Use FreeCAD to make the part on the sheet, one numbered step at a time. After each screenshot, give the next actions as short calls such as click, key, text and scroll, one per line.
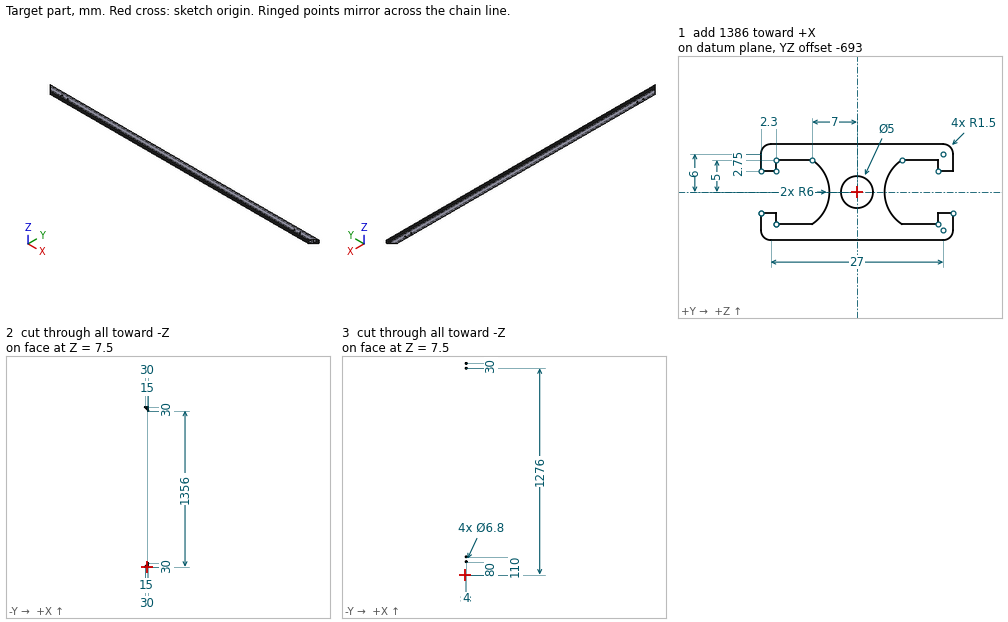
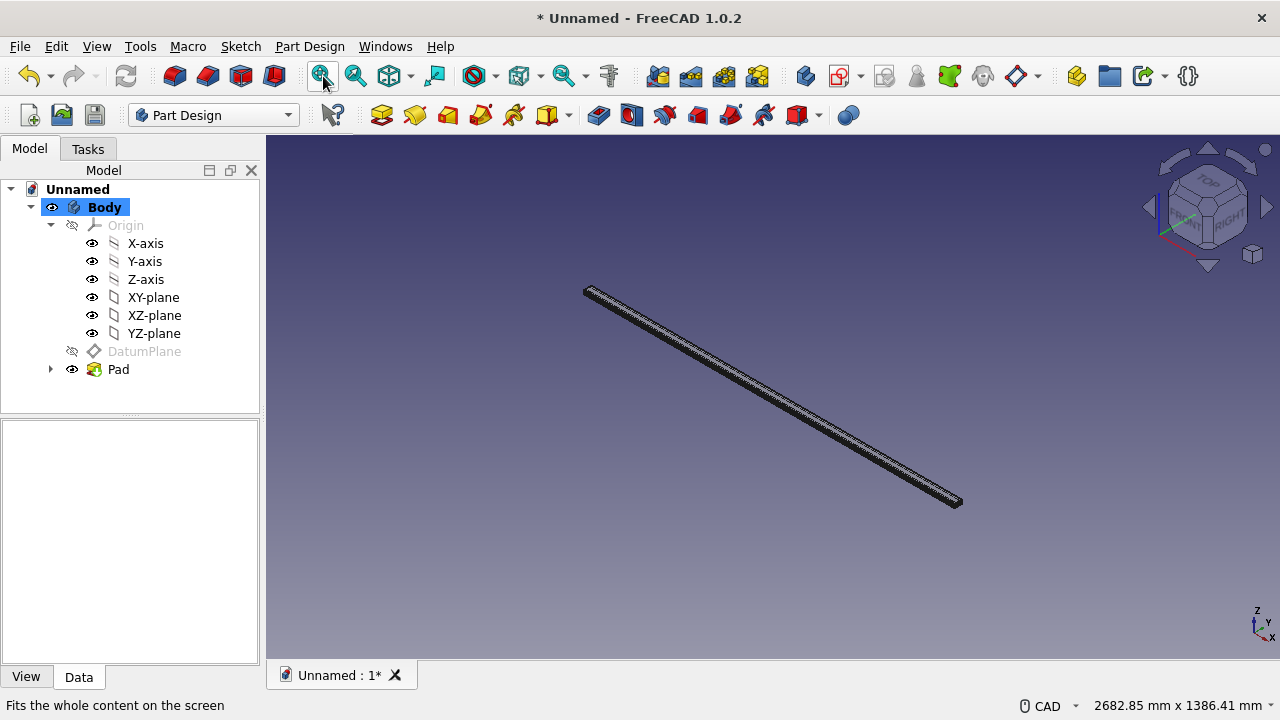
scroll(773, 394, up, 5)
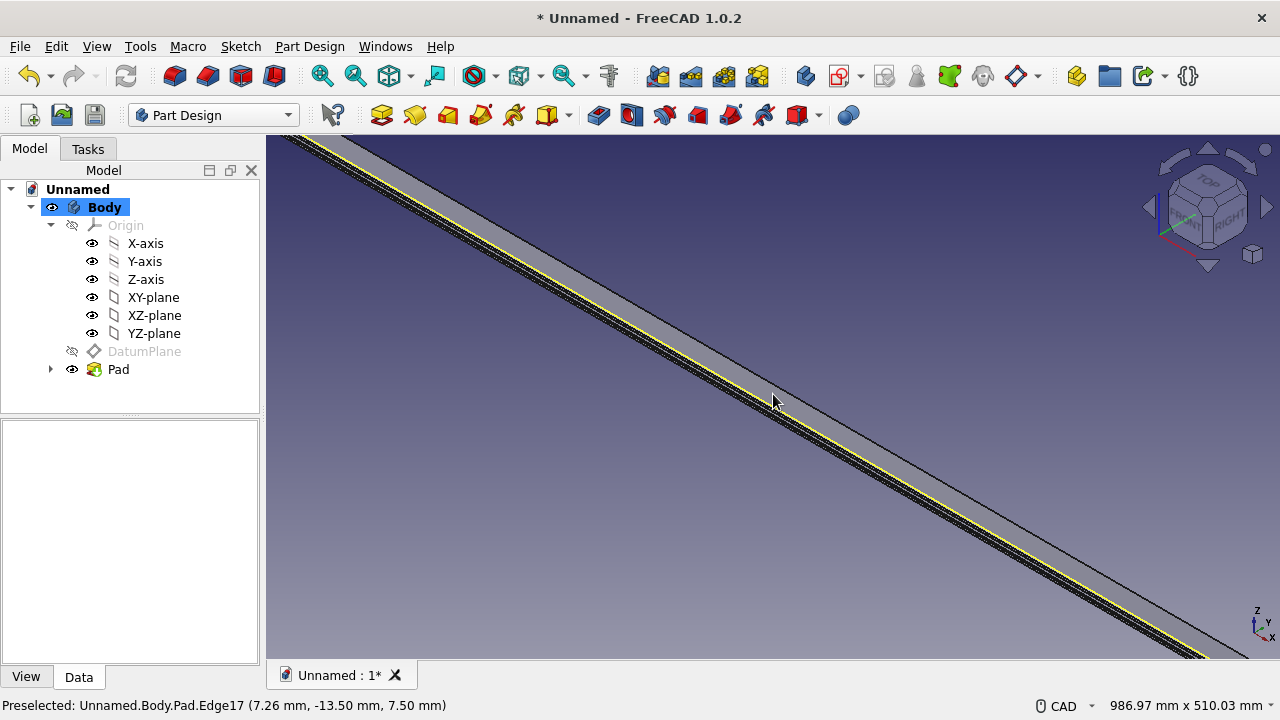
click(772, 394)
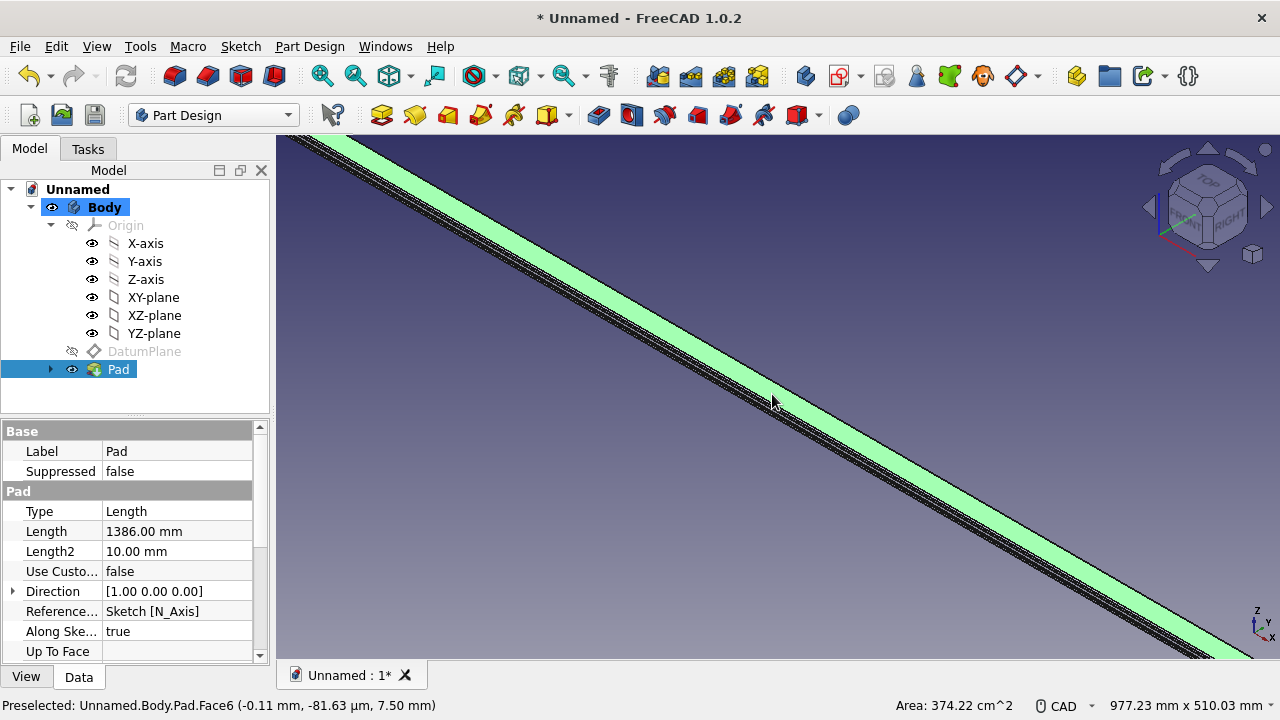
click(838, 76)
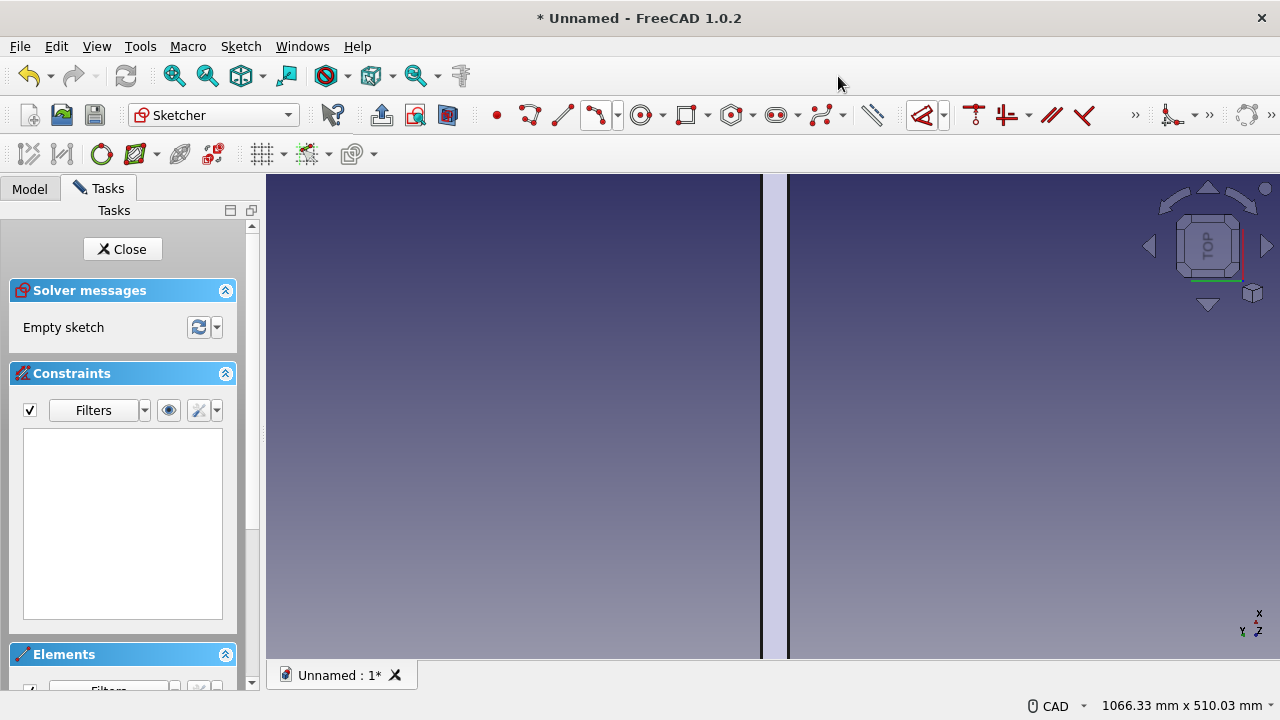
scroll(681, 417, down, 7)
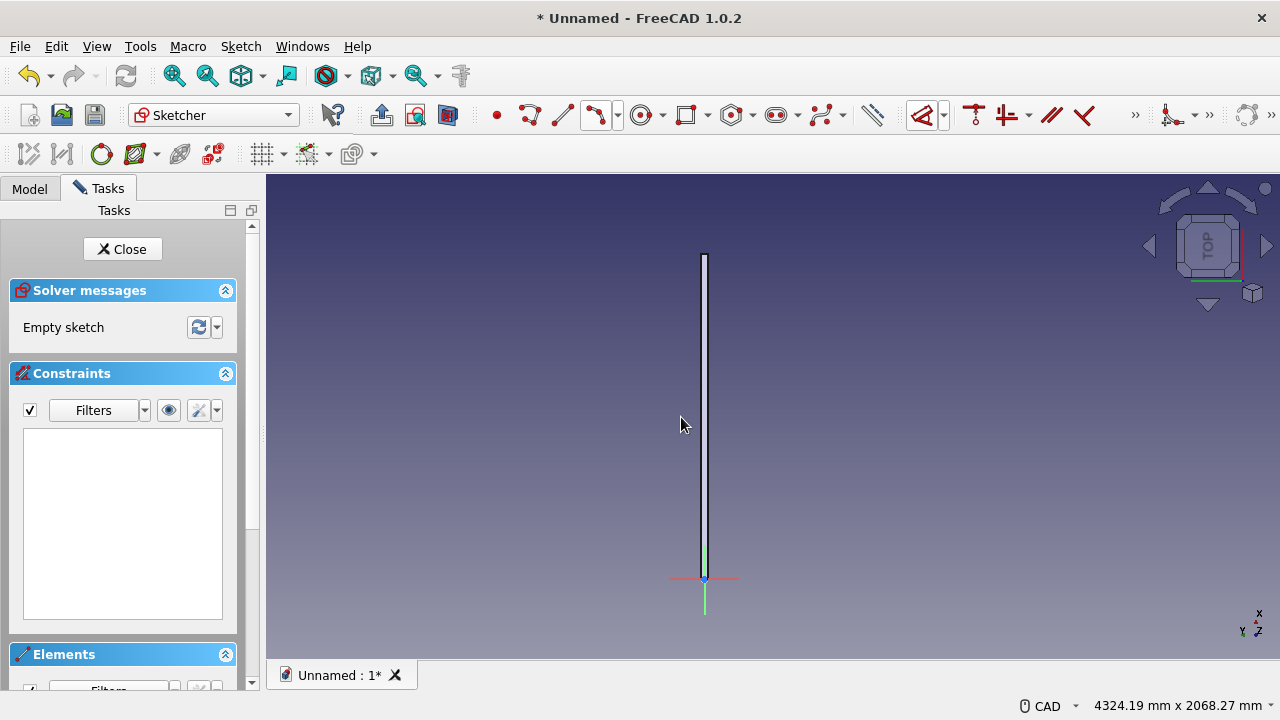
click(530, 116)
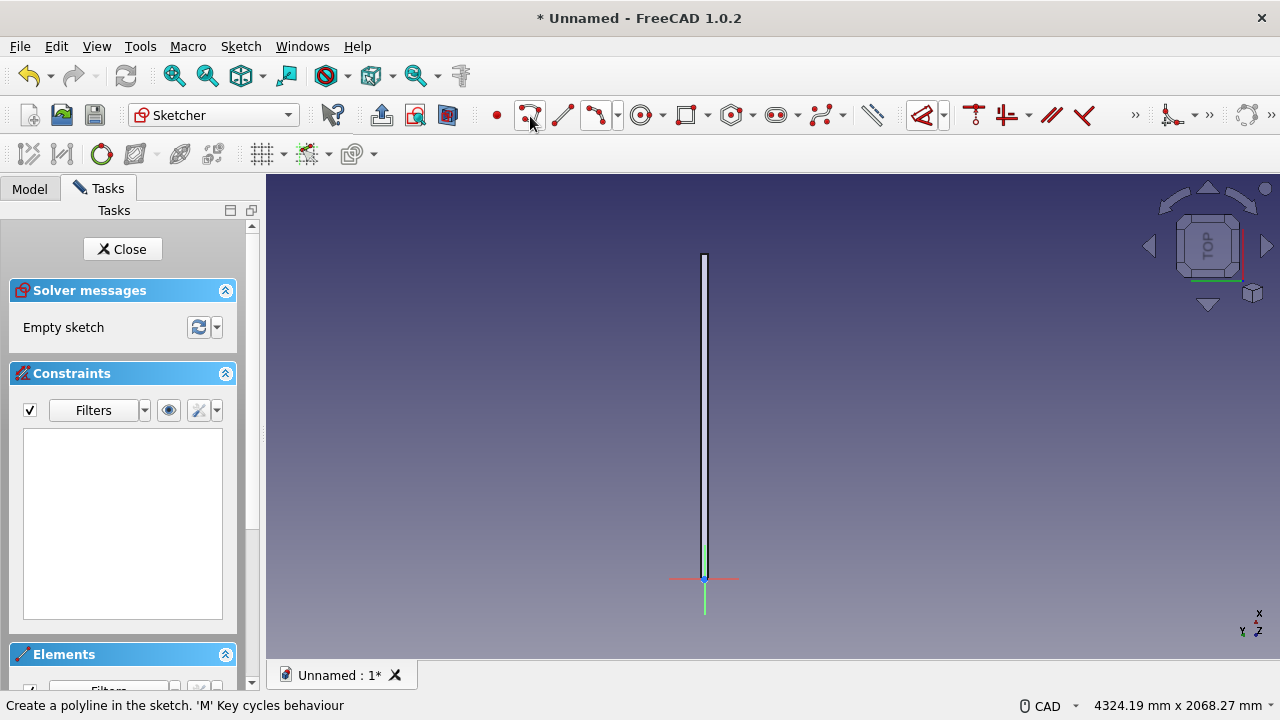
scroll(701, 579, up, 8)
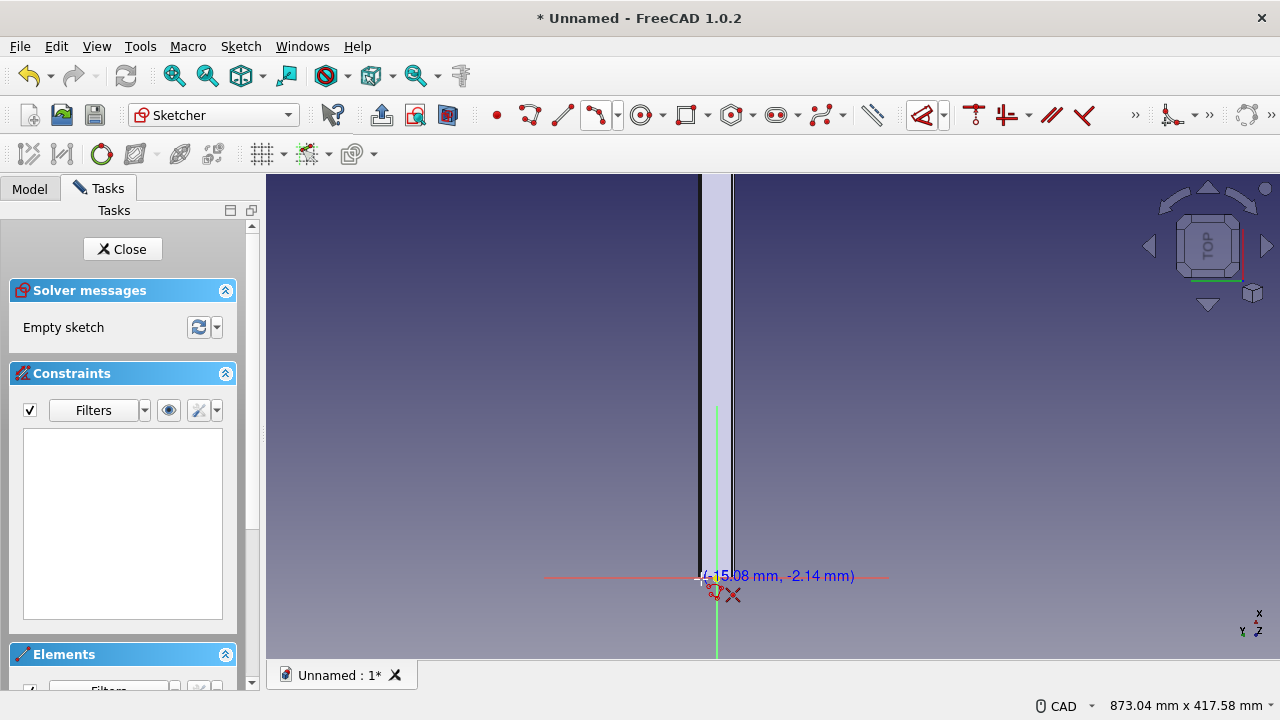
click(699, 578)
click(734, 569)
click(734, 543)
click(699, 578)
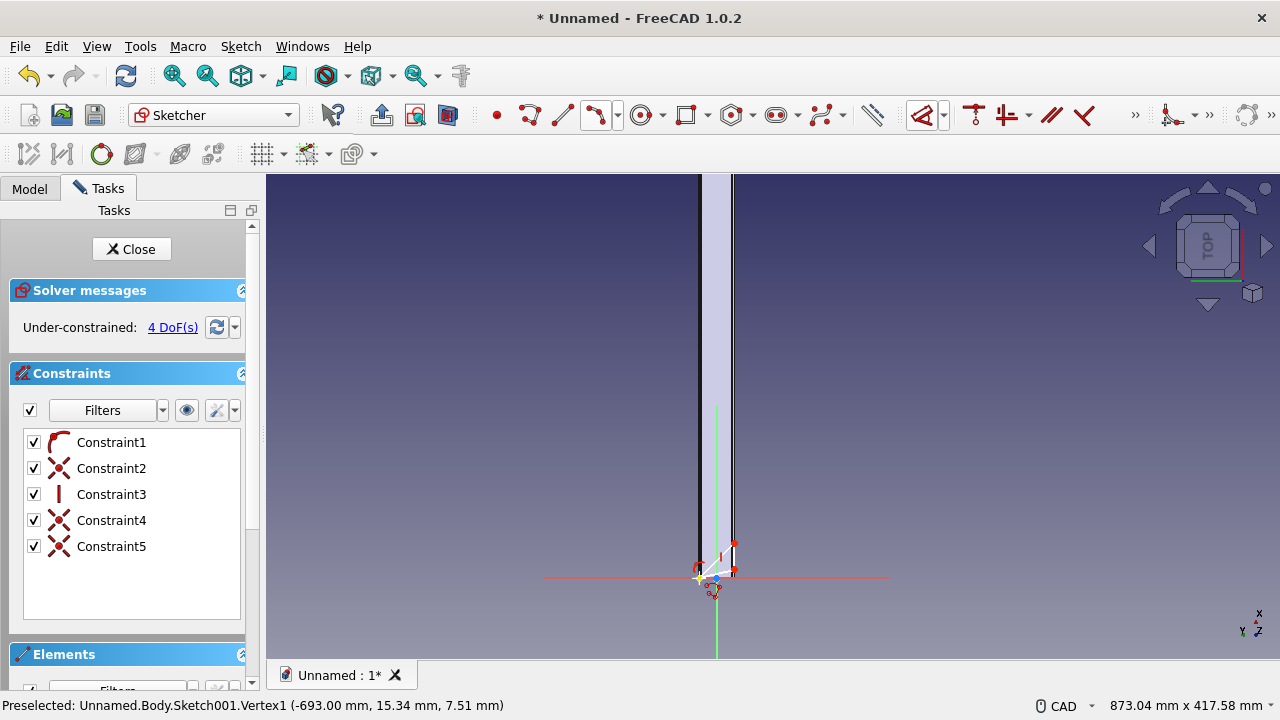
scroll(701, 579, down, 8)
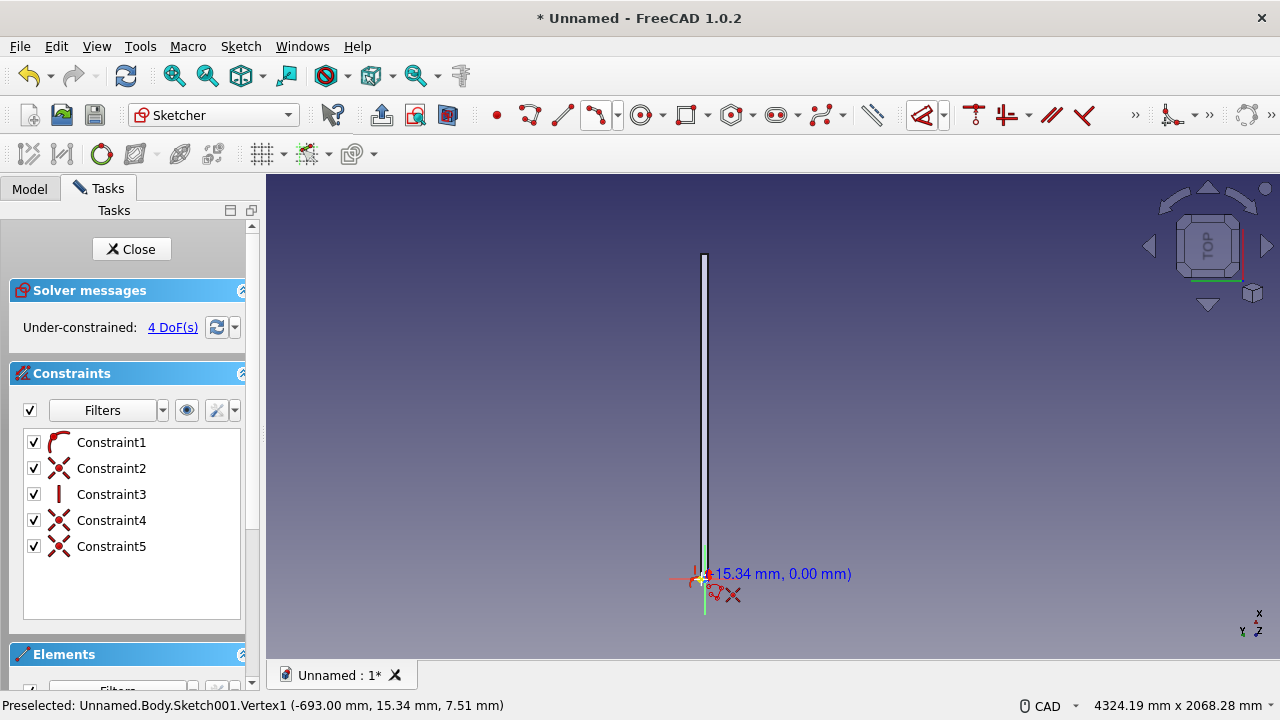
scroll(708, 262, up, 8)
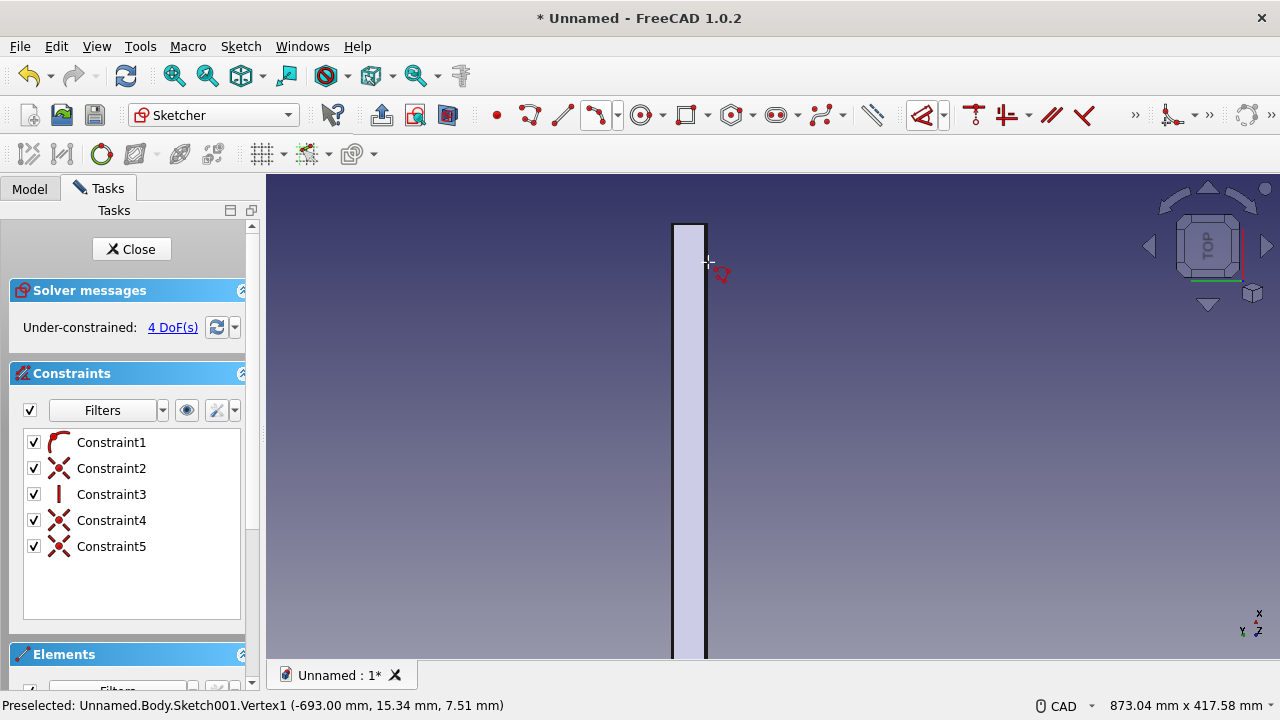
click(707, 259)
click(707, 224)
click(672, 224)
click(707, 260)
key(Escape)
key(Escape)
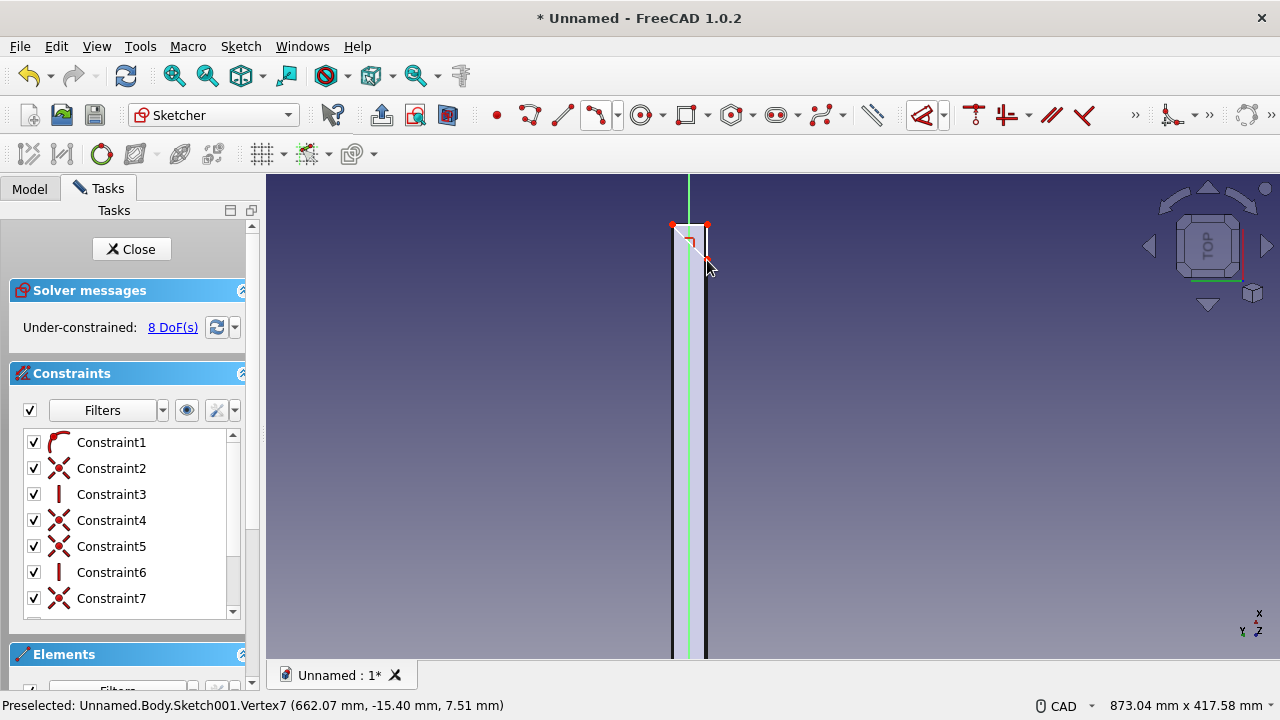
scroll(708, 262, down, 8)